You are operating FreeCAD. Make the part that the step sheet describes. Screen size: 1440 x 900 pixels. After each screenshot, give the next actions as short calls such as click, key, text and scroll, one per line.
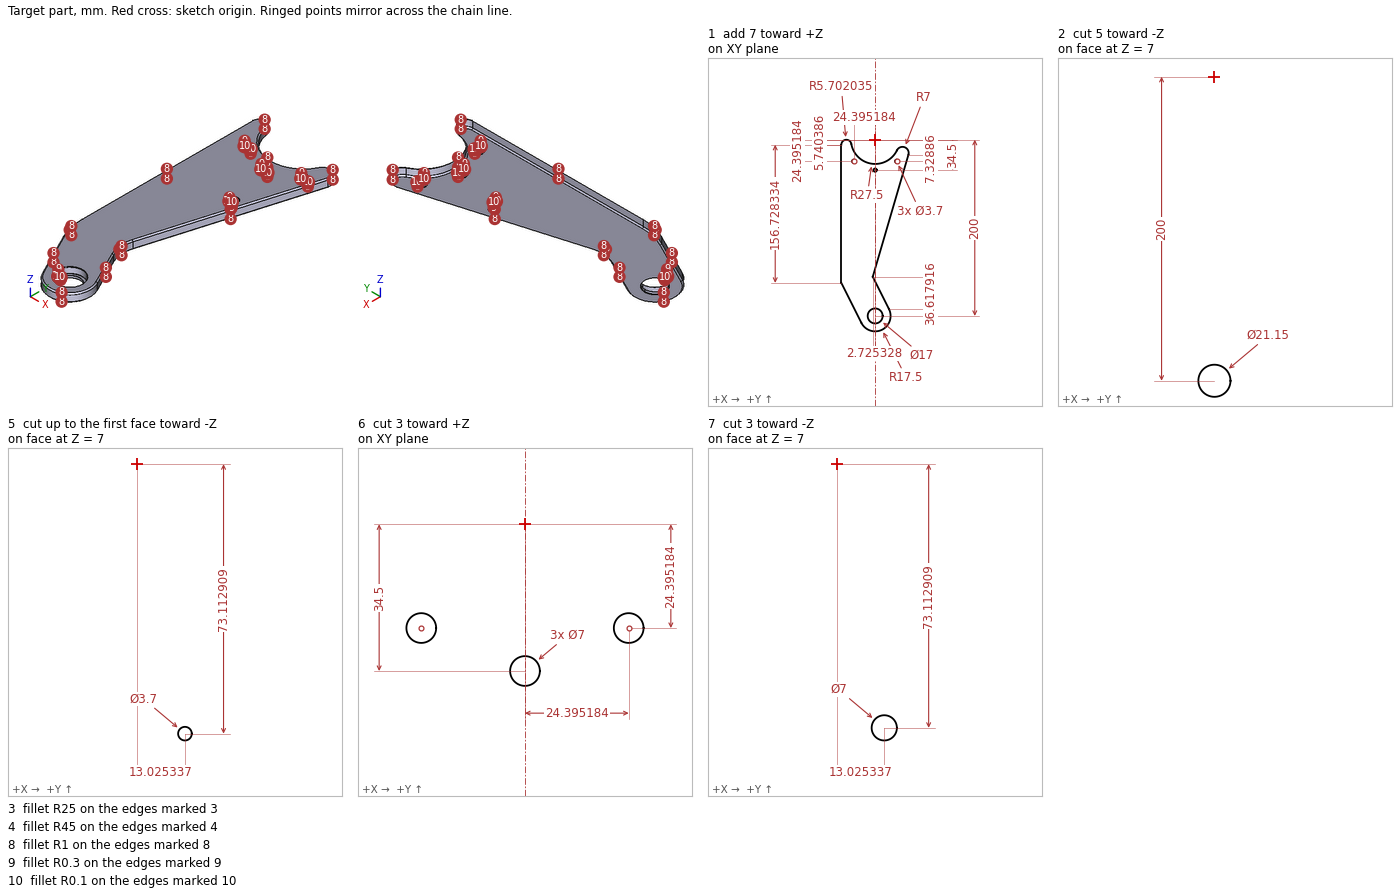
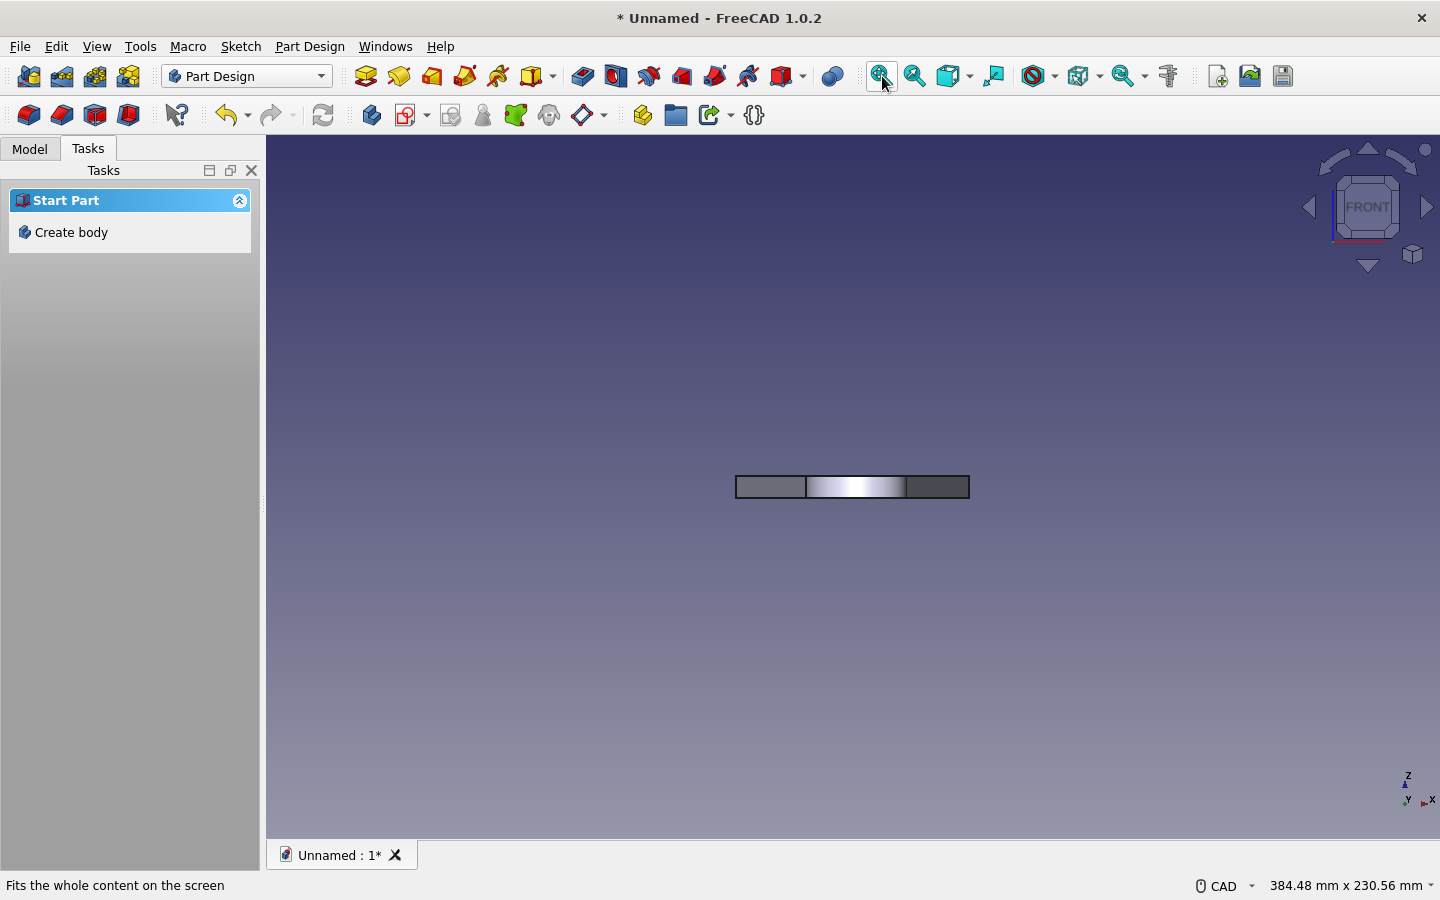
click(882, 76)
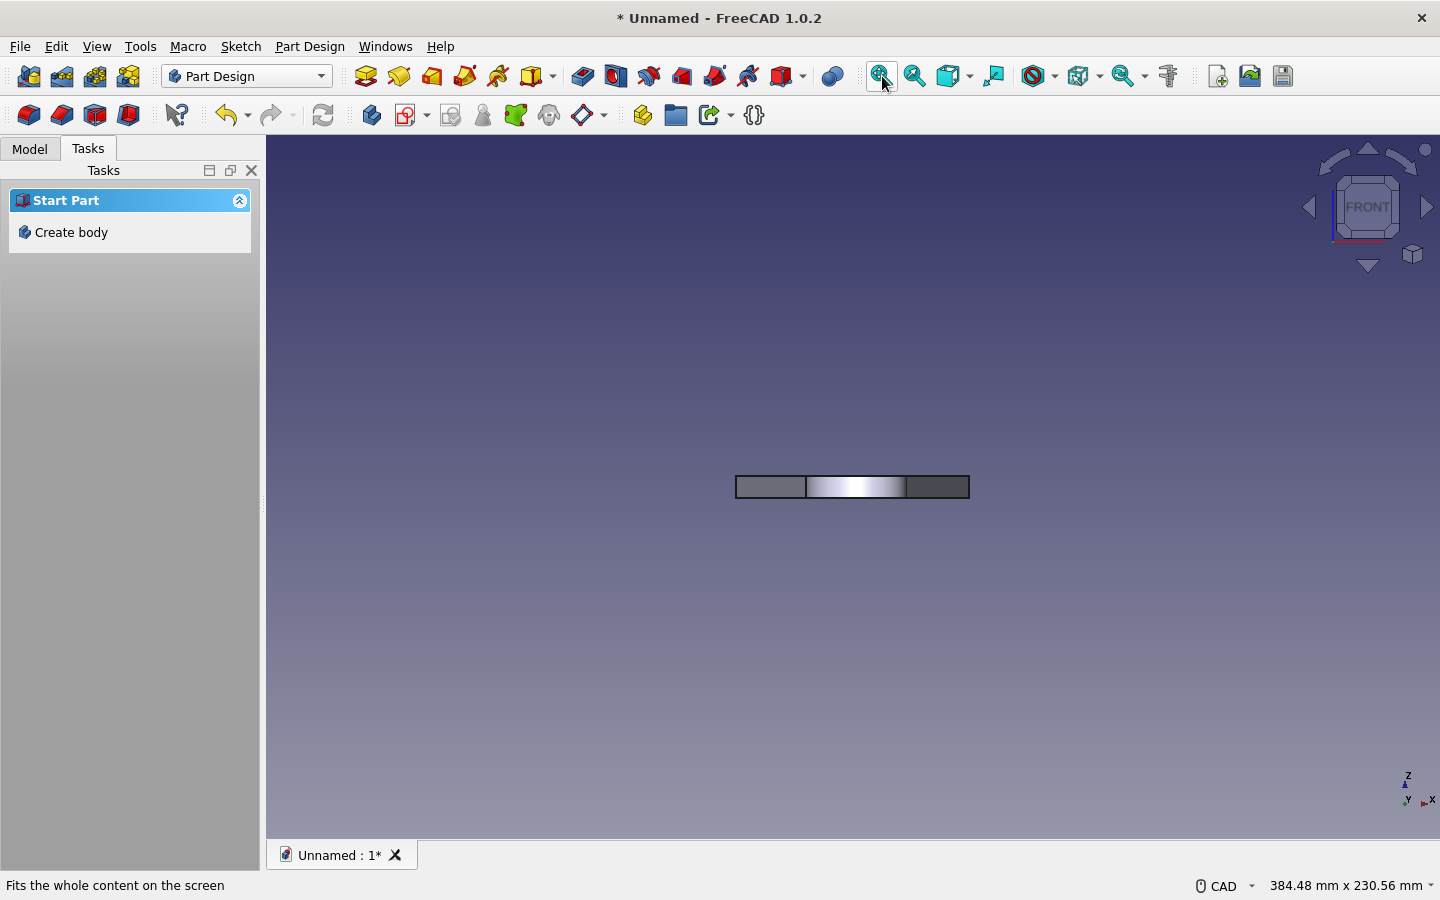
scroll(736, 486, up, 4)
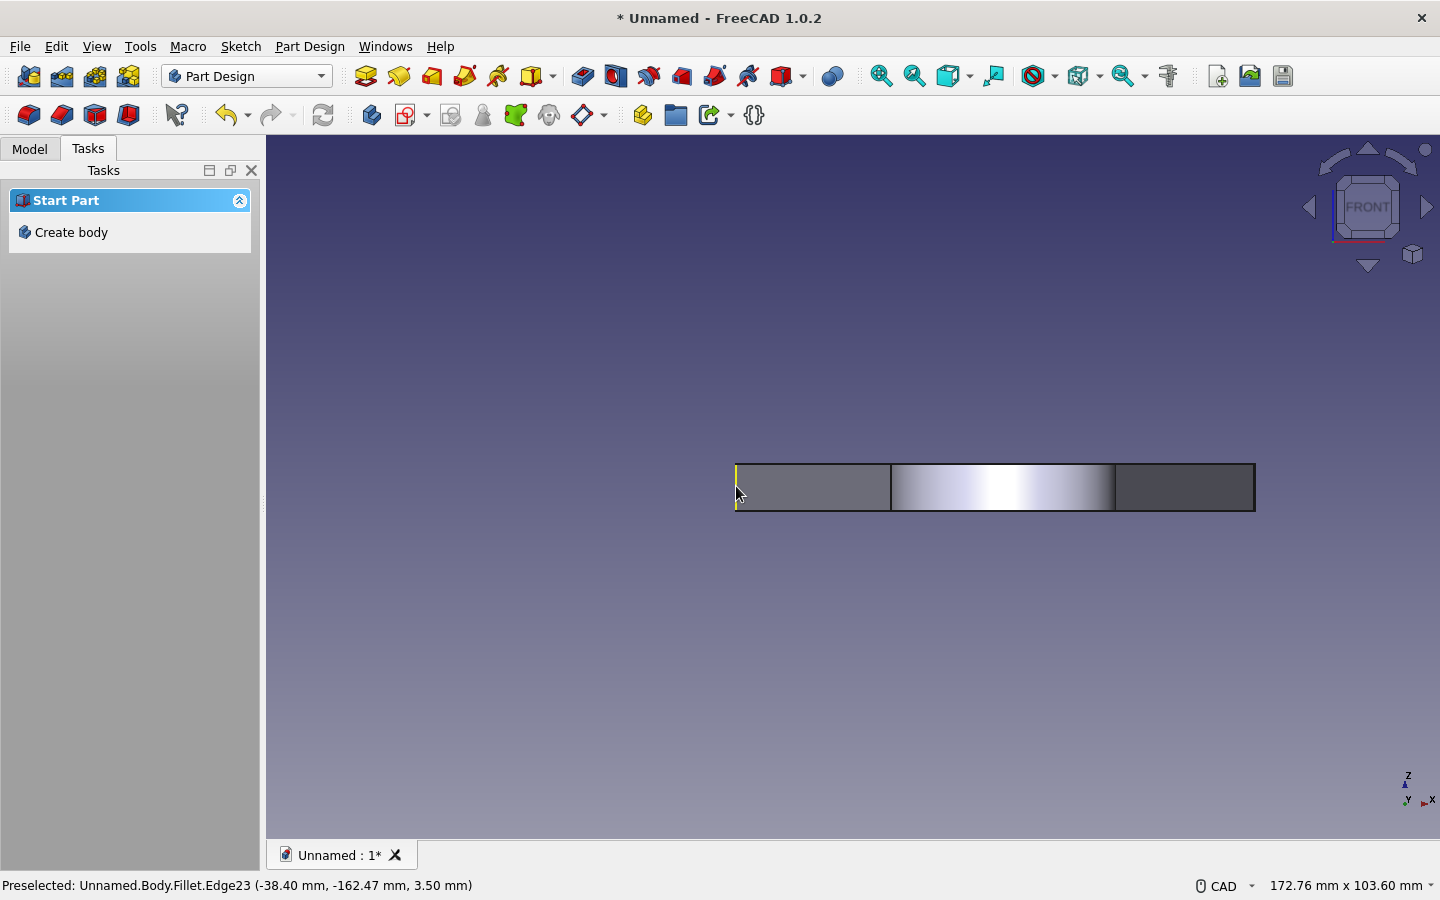
click(882, 76)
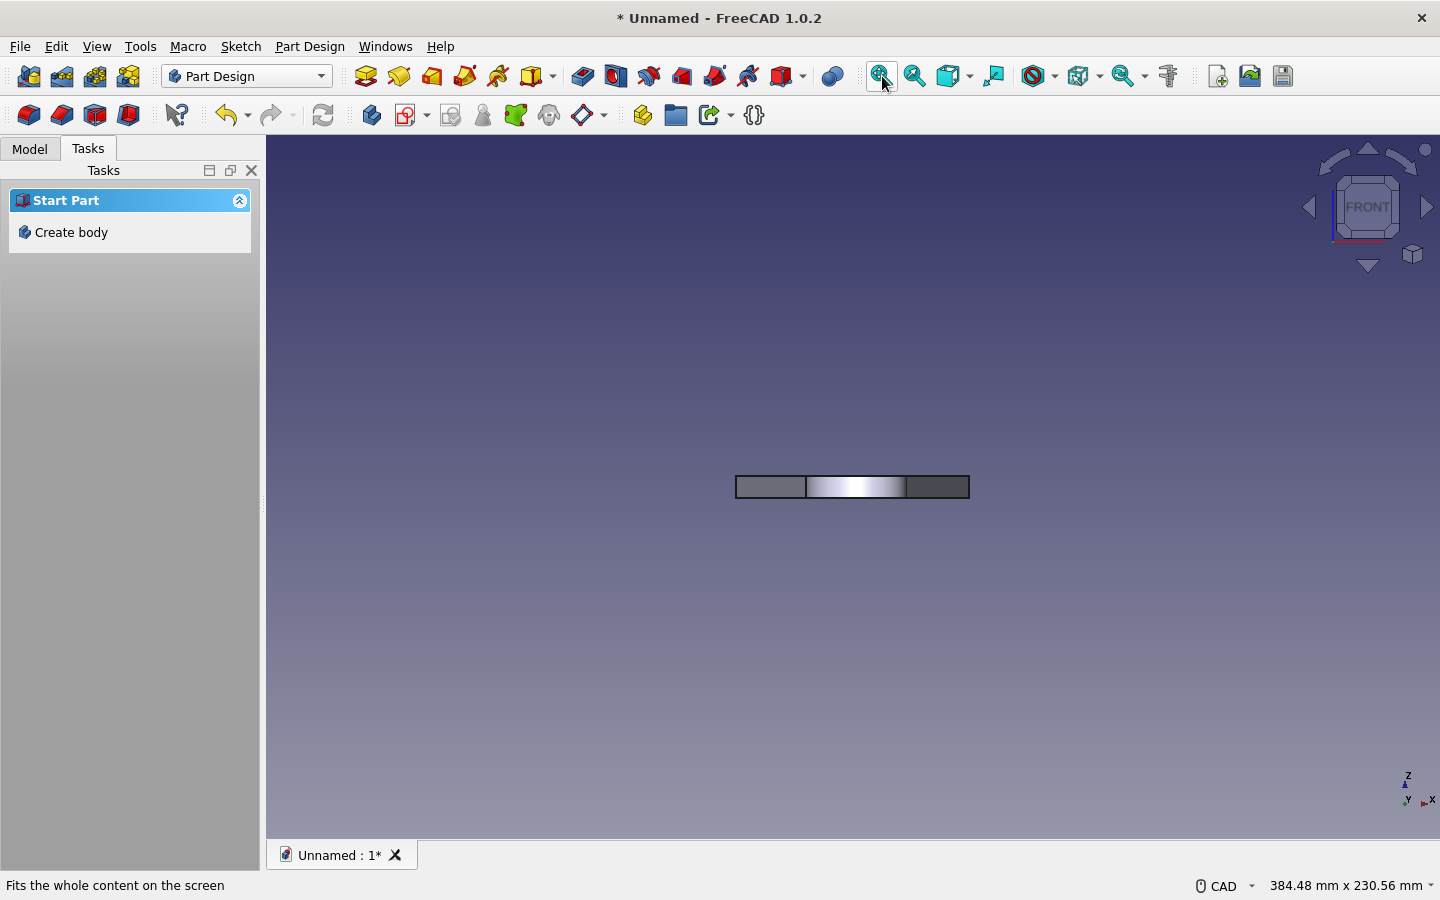
key(3)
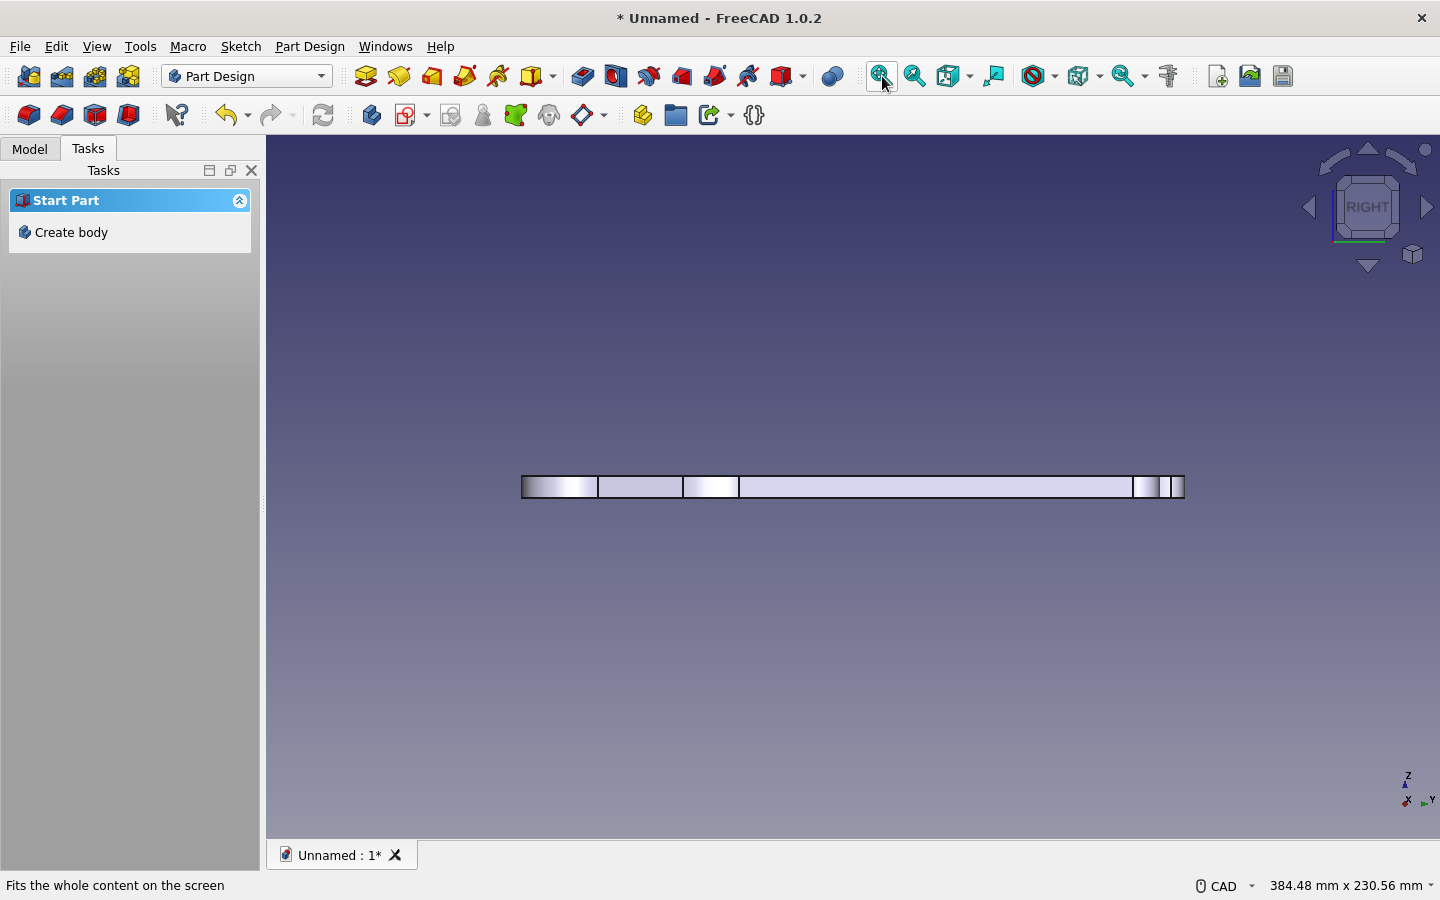
scroll(689, 486, up, 4)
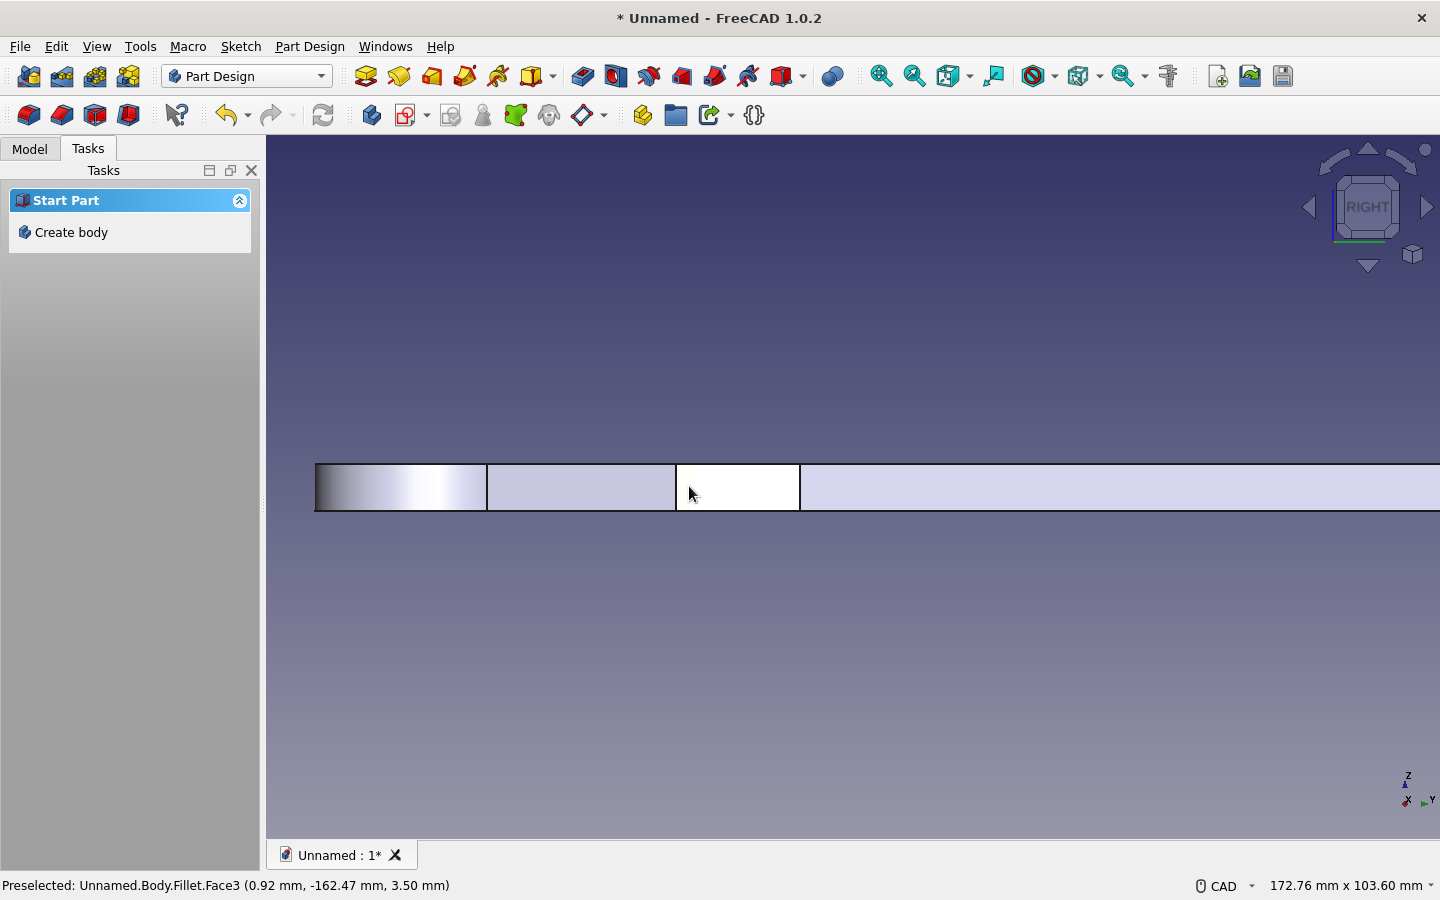
click(882, 76)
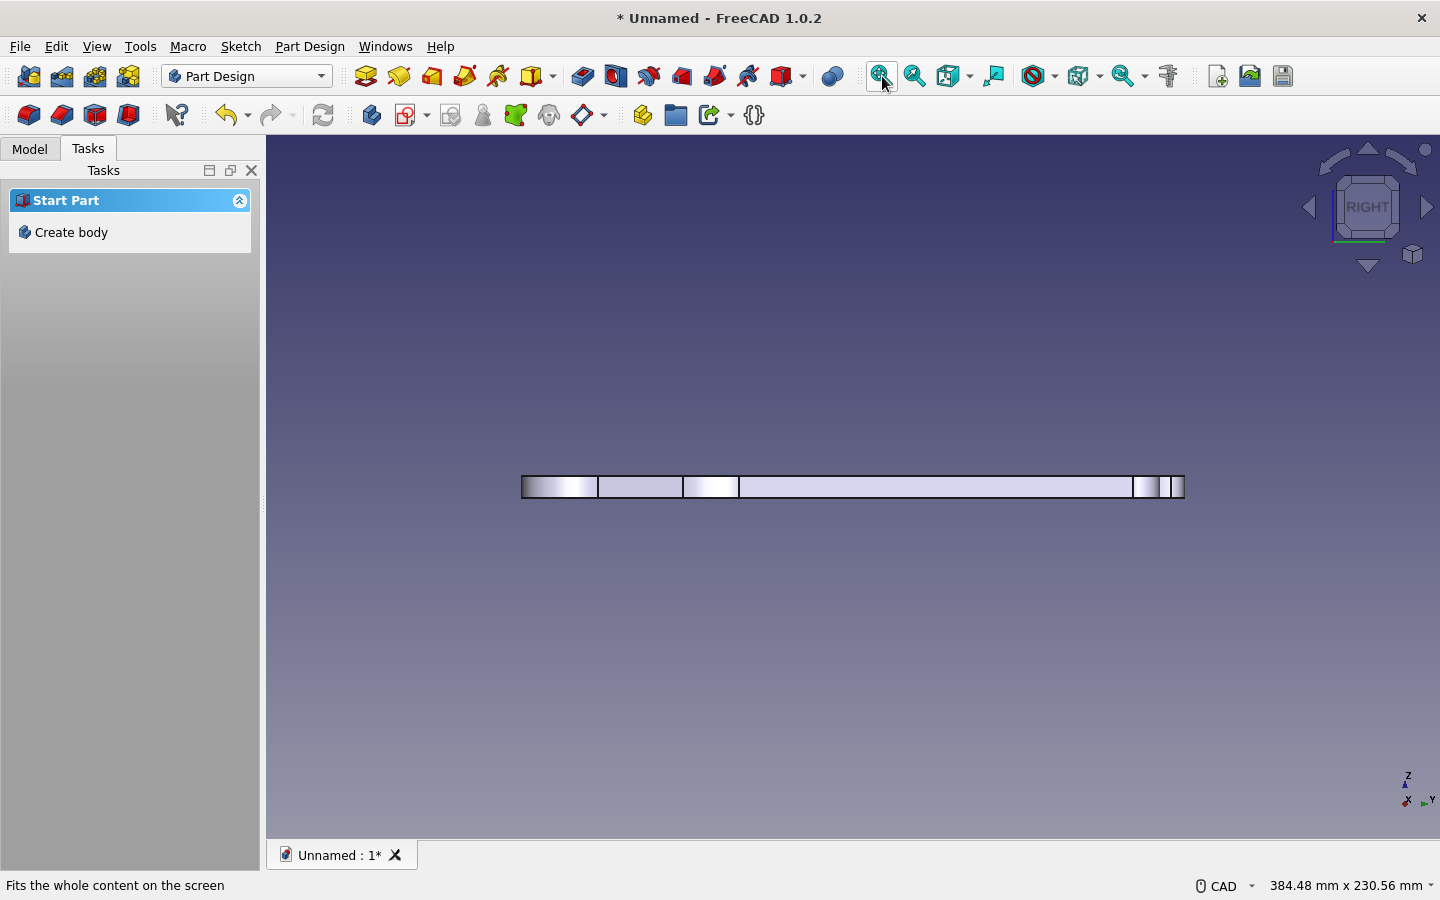
key(5)